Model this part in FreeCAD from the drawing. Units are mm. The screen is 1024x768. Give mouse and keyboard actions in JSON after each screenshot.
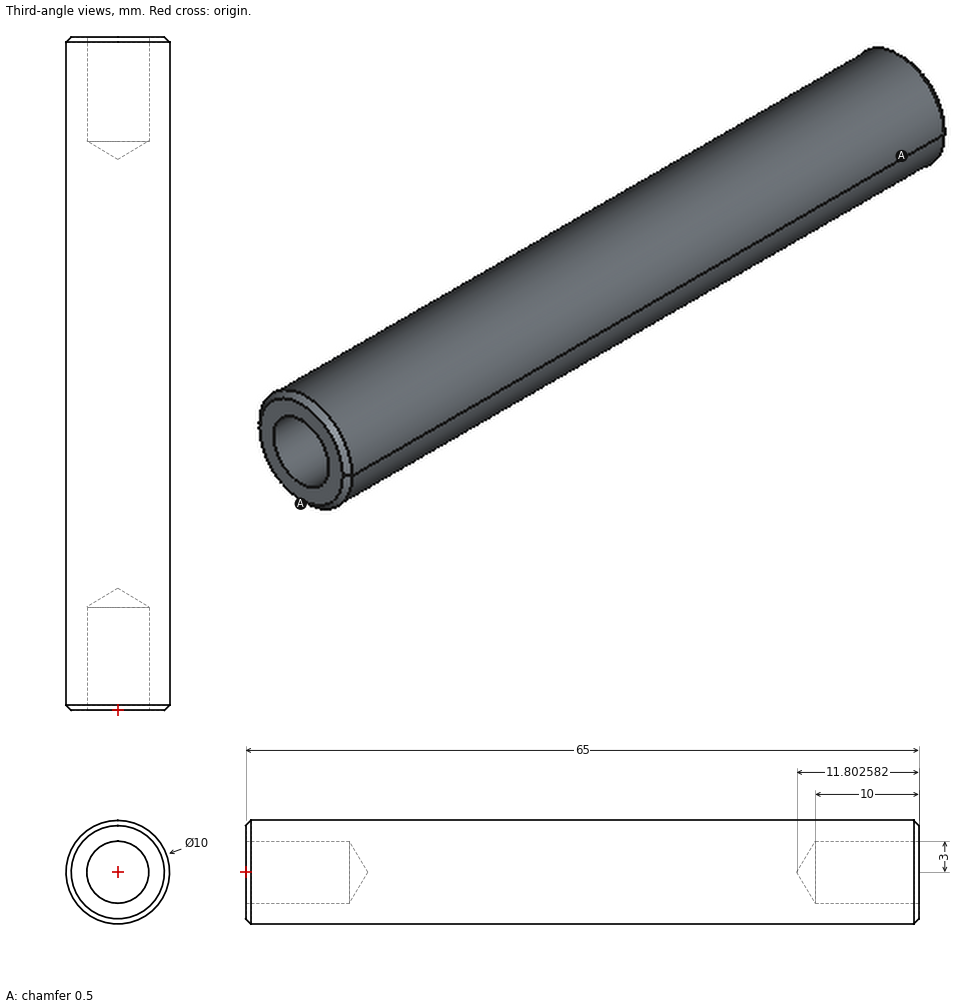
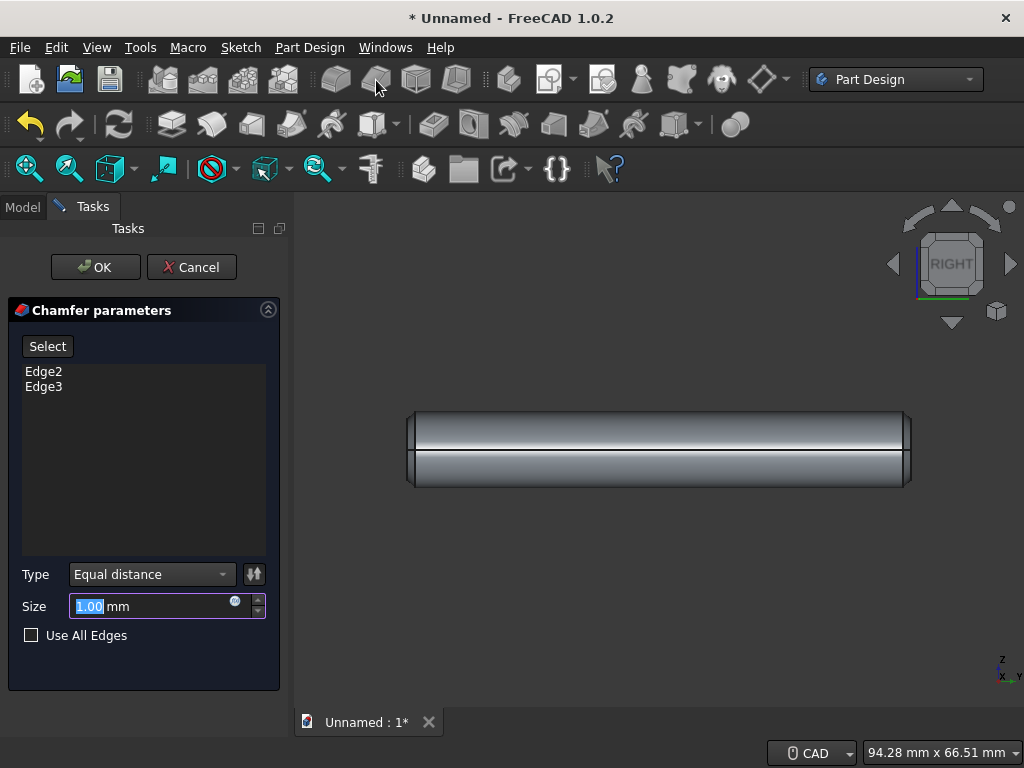
{"action": "type", "text": "0.5"}
{"action": "key", "text": "Tab"}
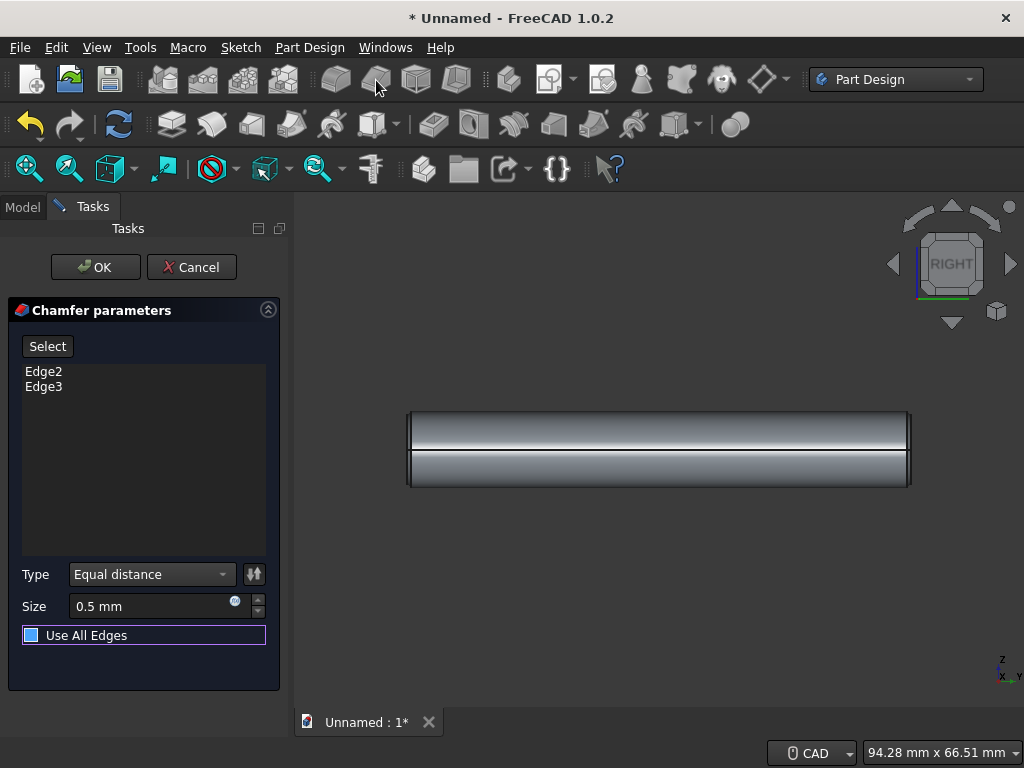
{"action": "left_click", "coordinate": [96, 267]}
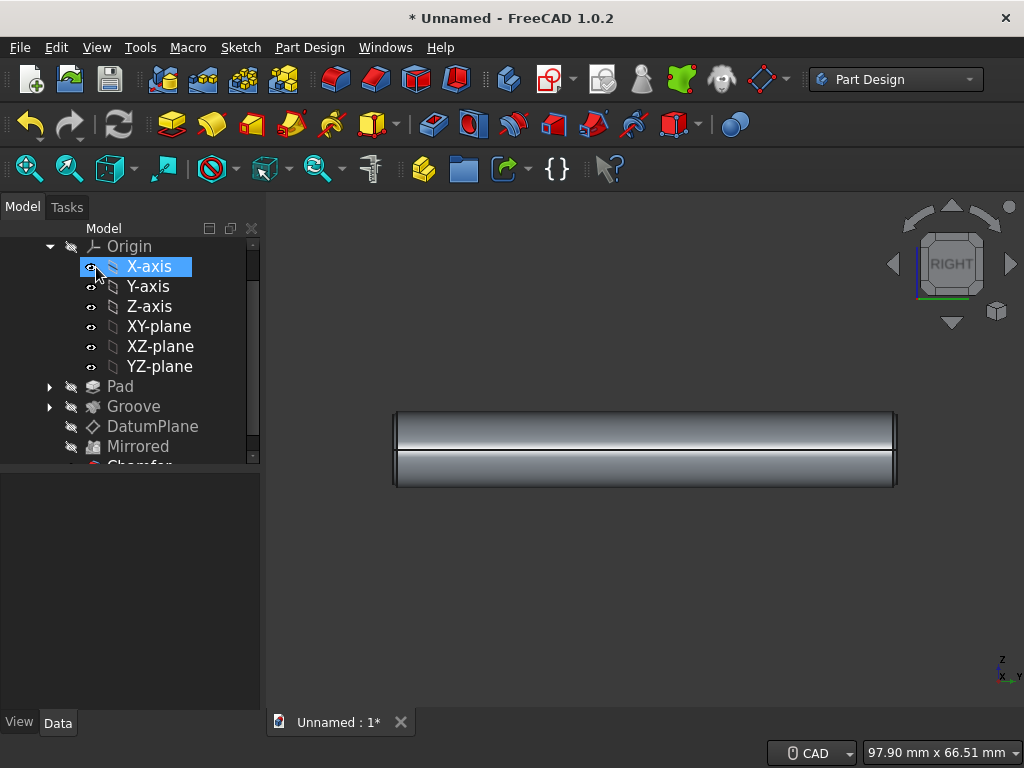
{"action": "key", "text": "0"}